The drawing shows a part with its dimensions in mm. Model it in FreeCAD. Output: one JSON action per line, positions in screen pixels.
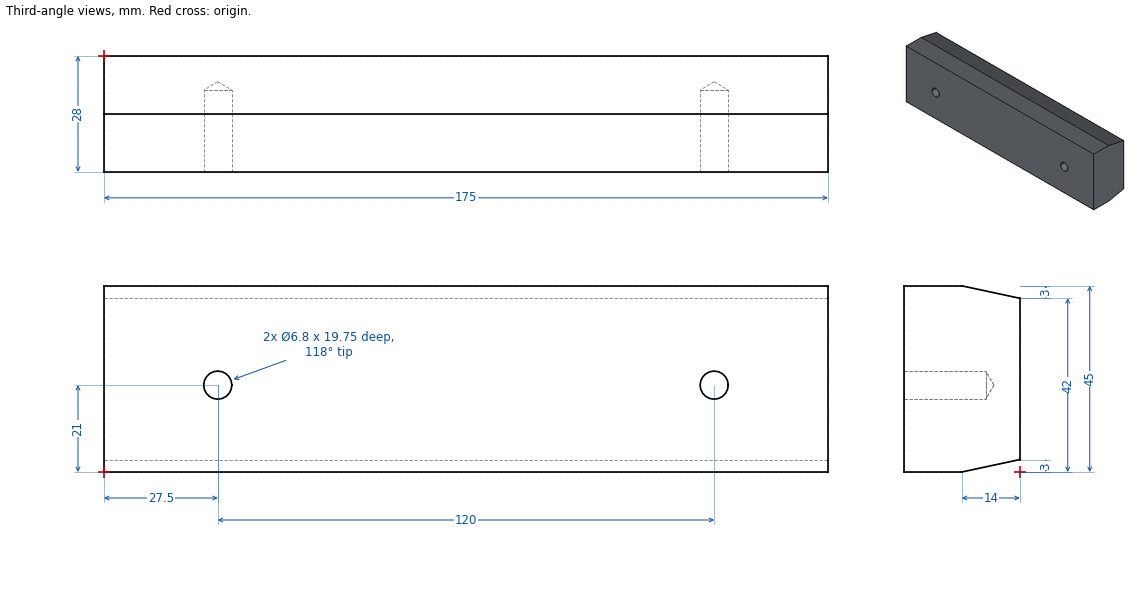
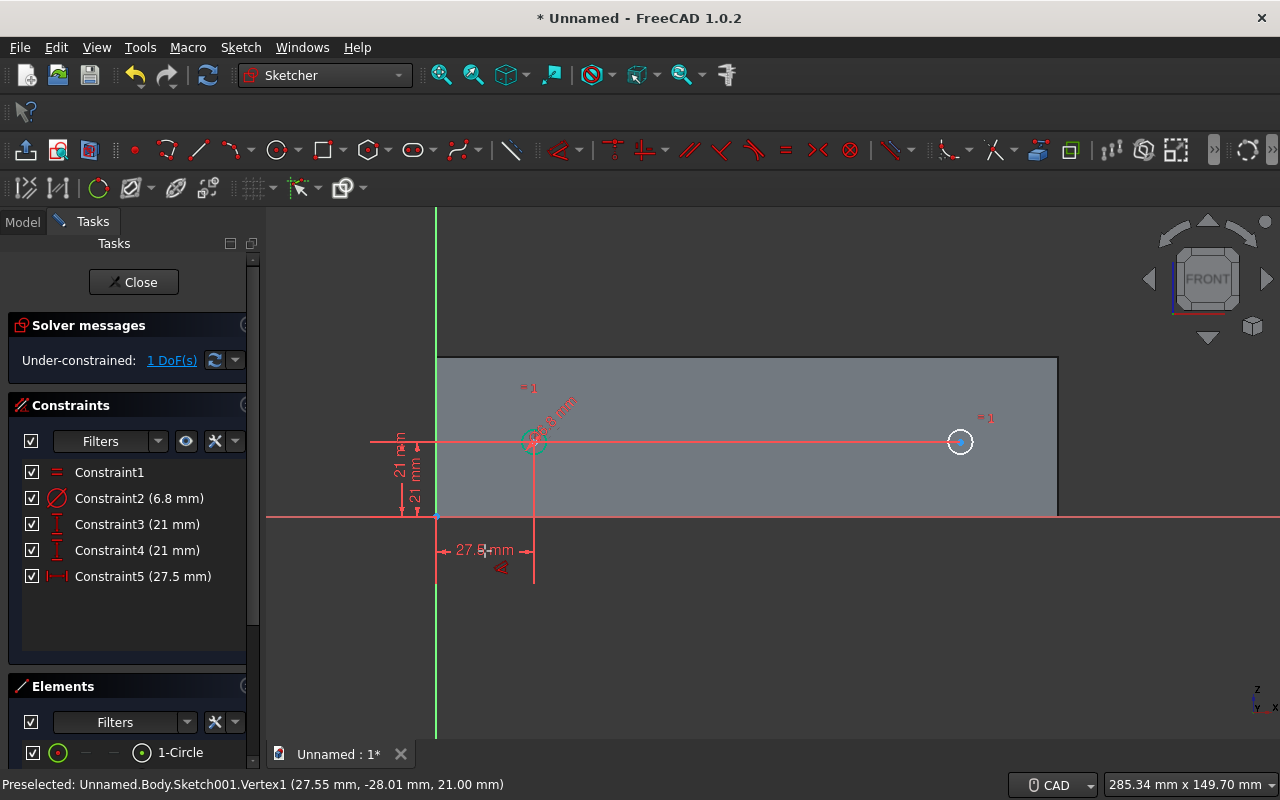
{"action": "left_click", "coordinate": [534, 442]}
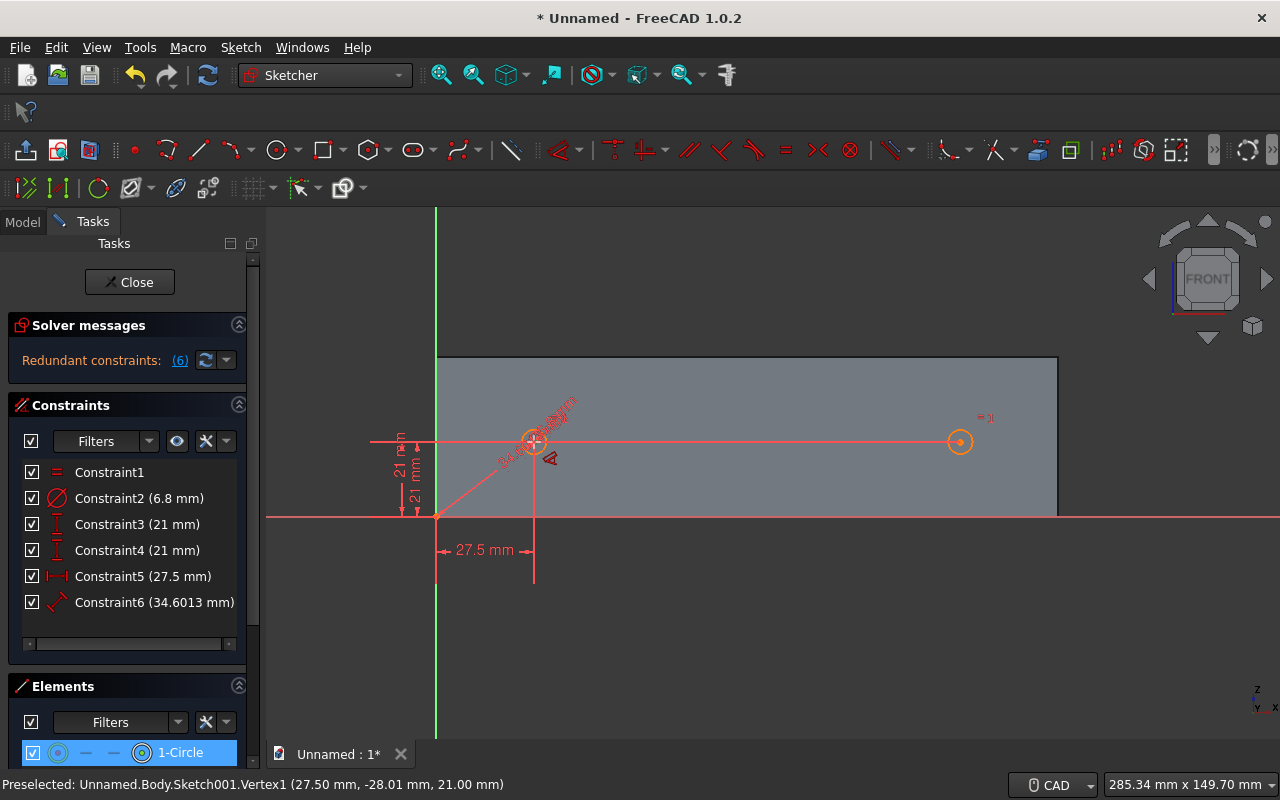
{"action": "left_click", "coordinate": [960, 442]}
{"action": "left_click", "coordinate": [747, 408]}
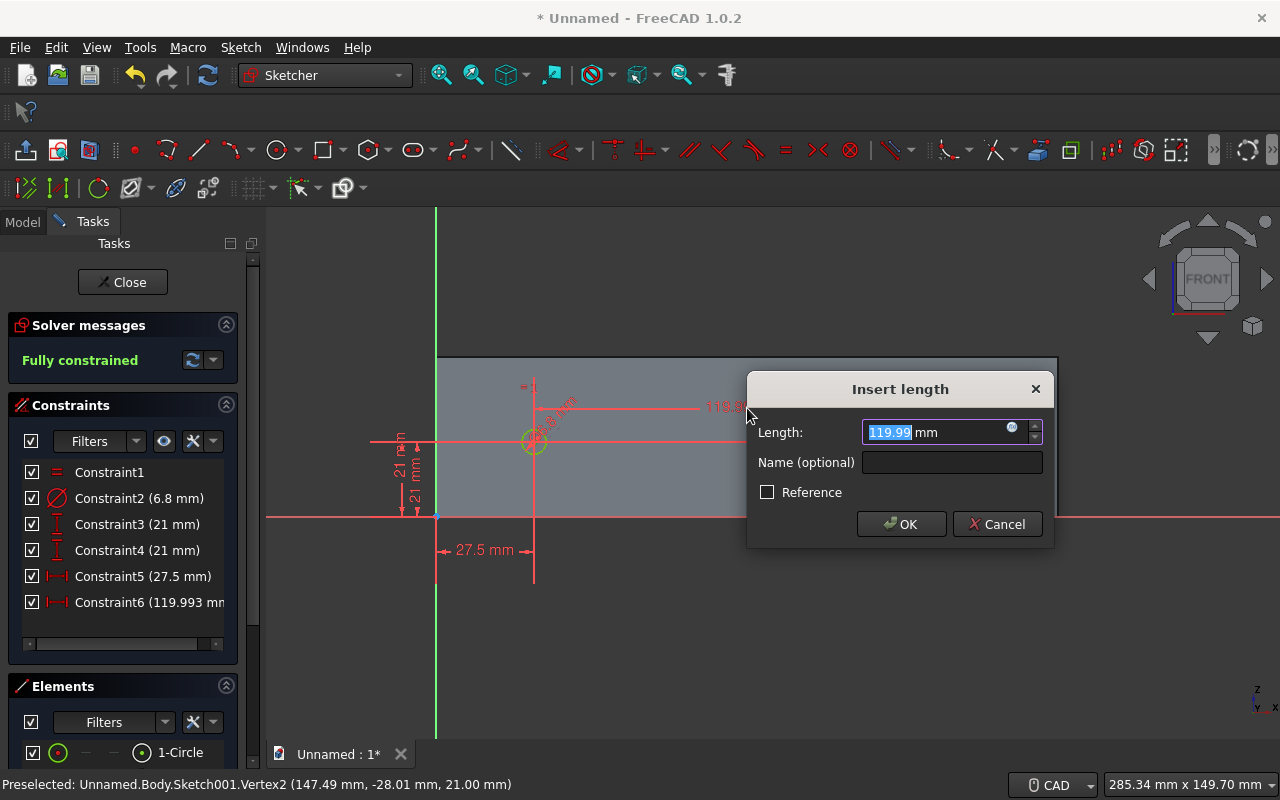
{"action": "type", "text": "120"}
{"action": "key", "text": "Return"}
{"action": "key", "text": "Escape"}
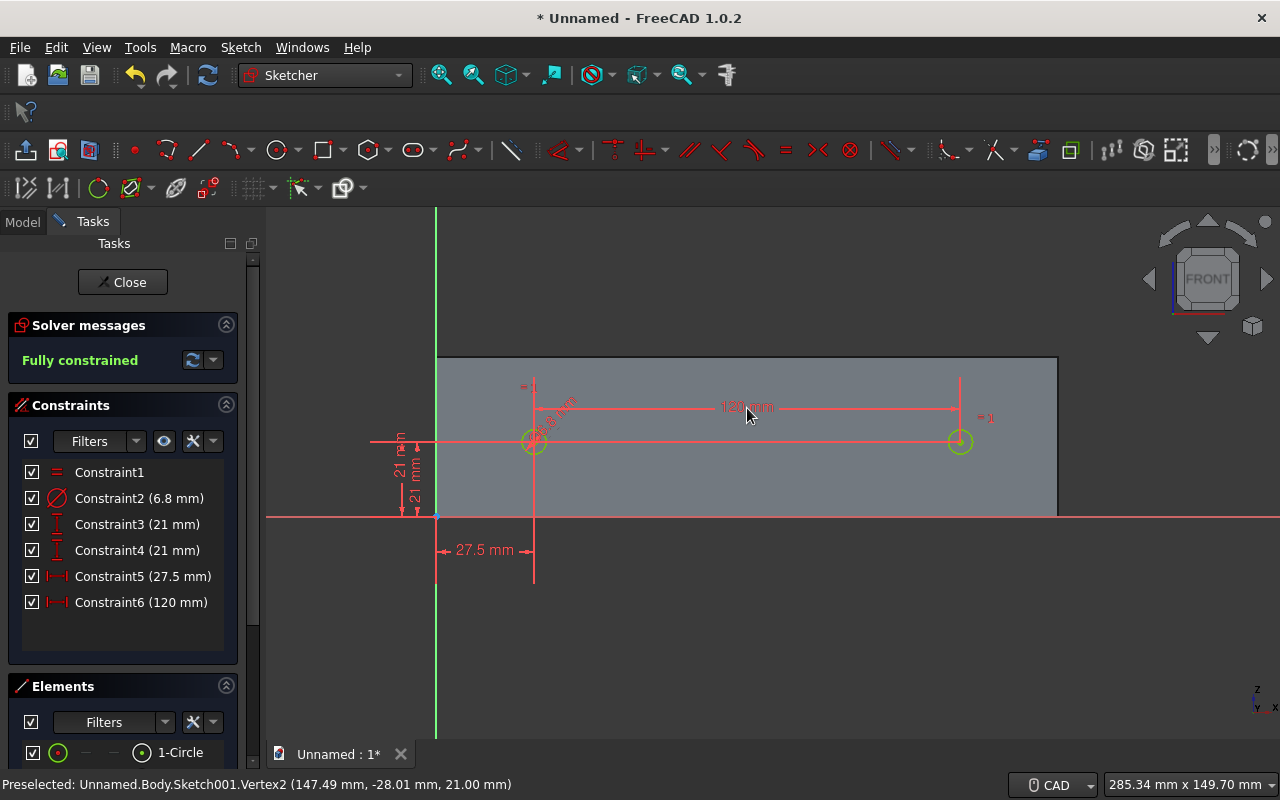
{"action": "left_click", "coordinate": [123, 282]}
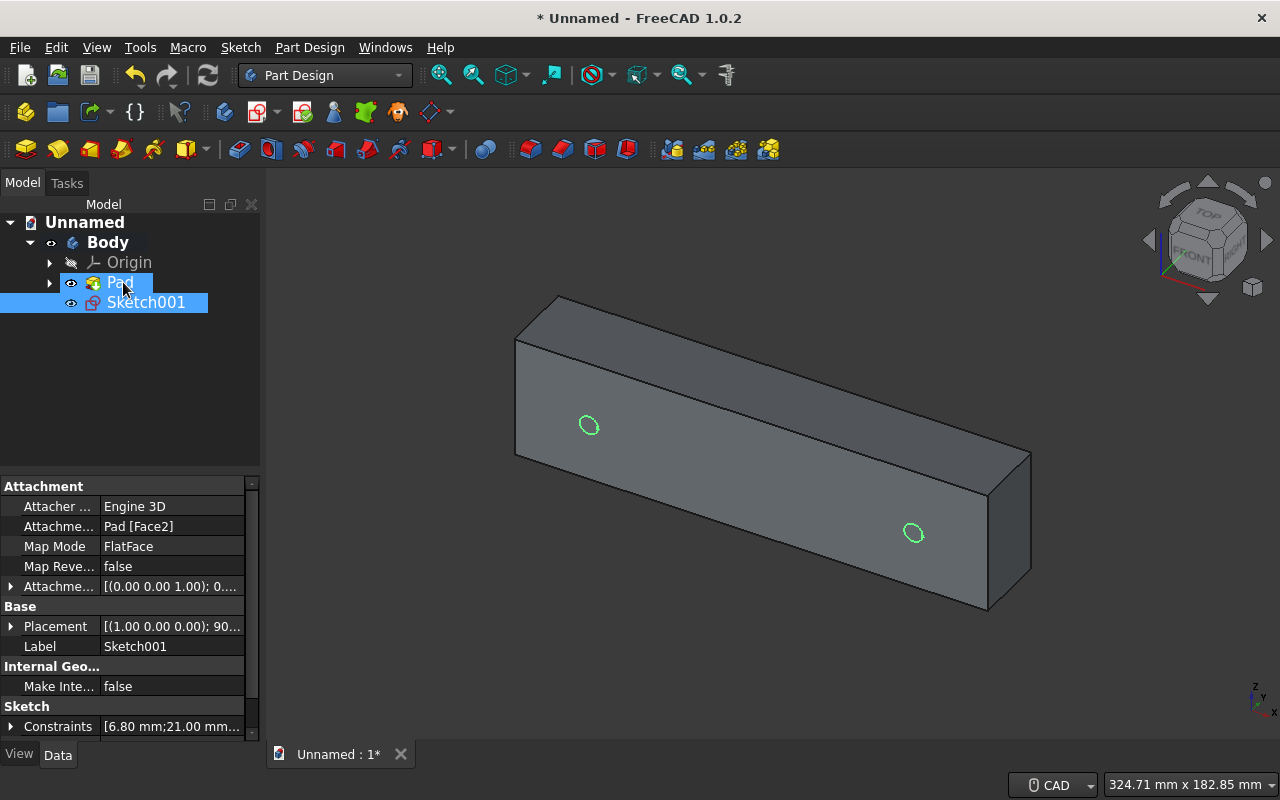
{"action": "left_click", "coordinate": [272, 150]}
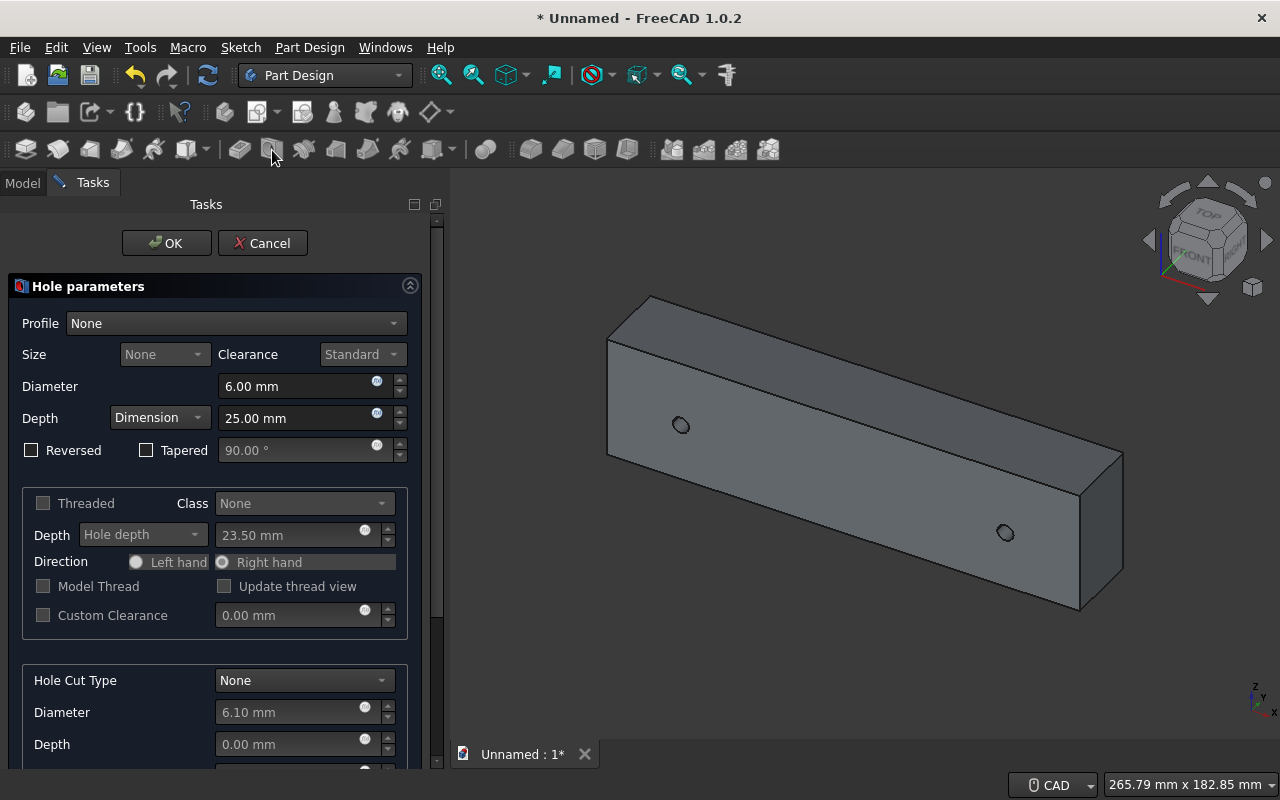
{"action": "triple_click", "coordinate": [305, 386]}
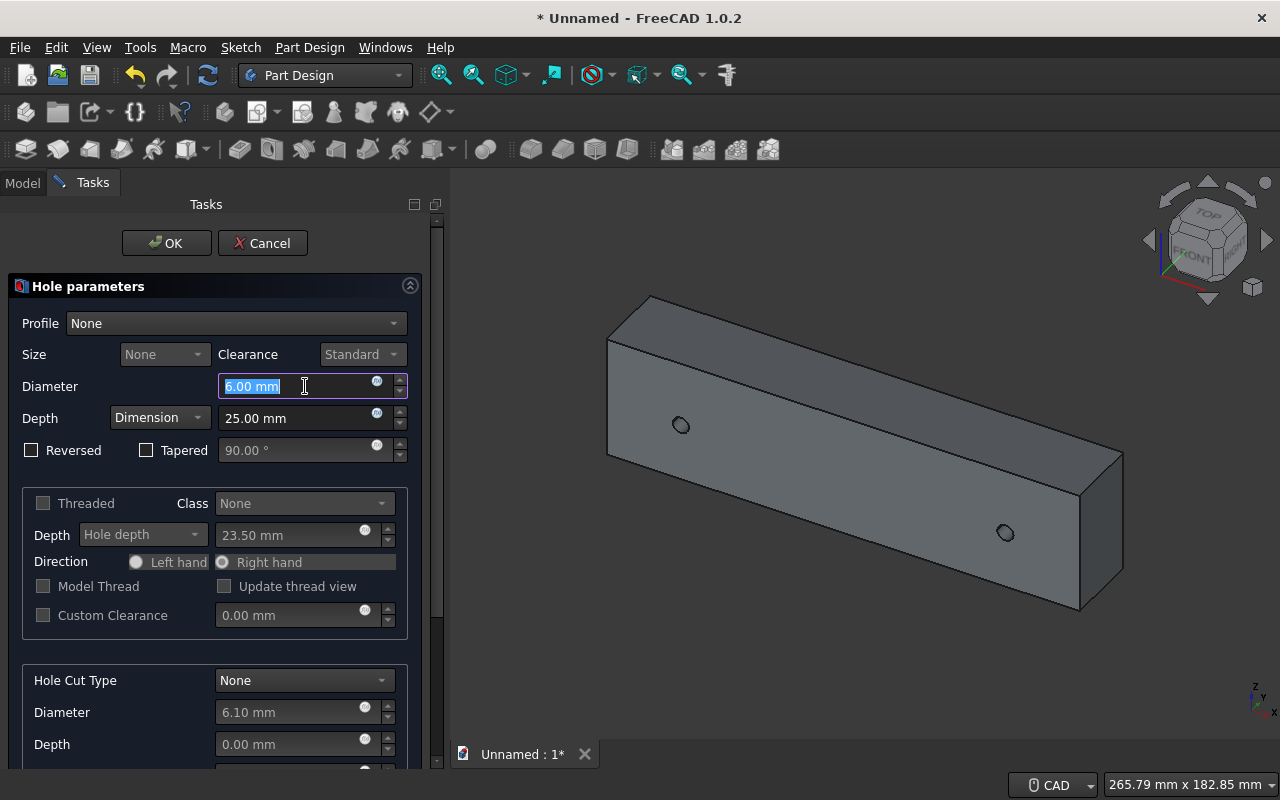
{"action": "type", "text": "6.8"}
{"action": "key", "text": "Tab"}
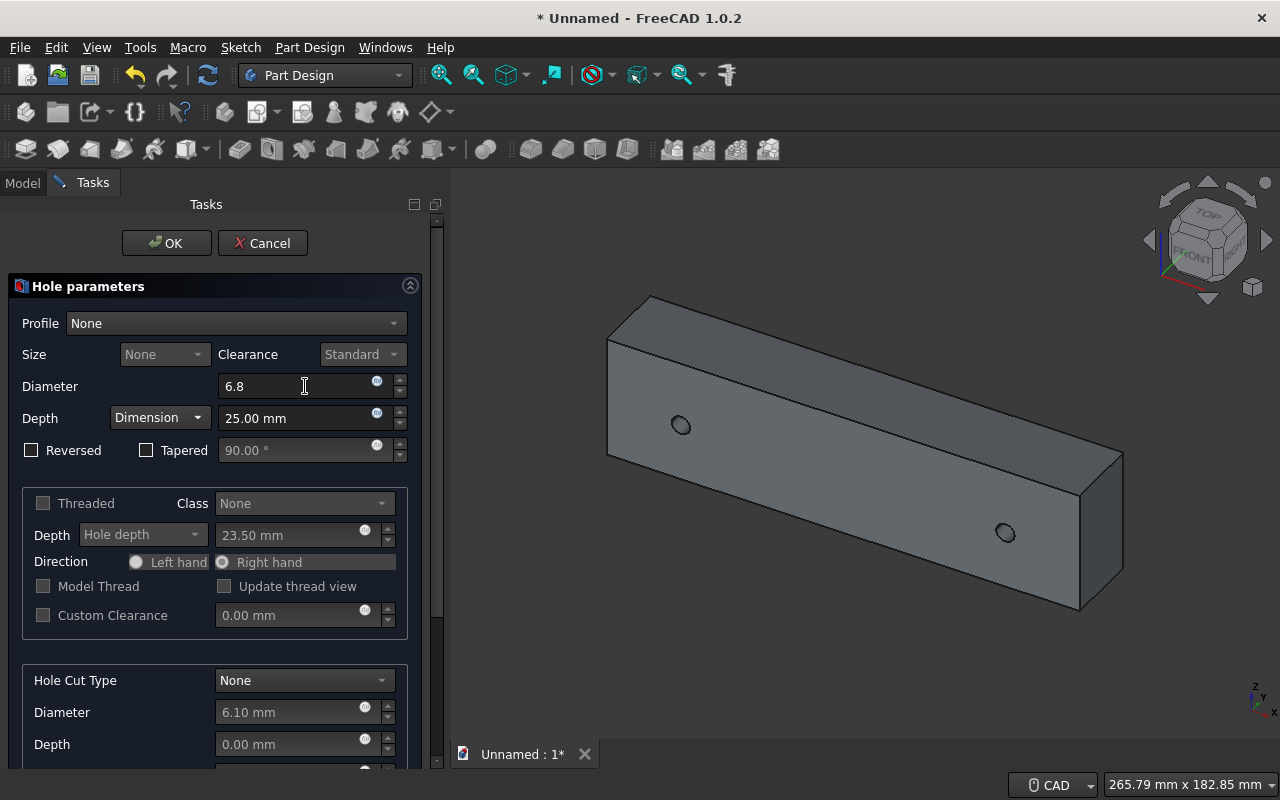
{"action": "triple_click", "coordinate": [305, 418]}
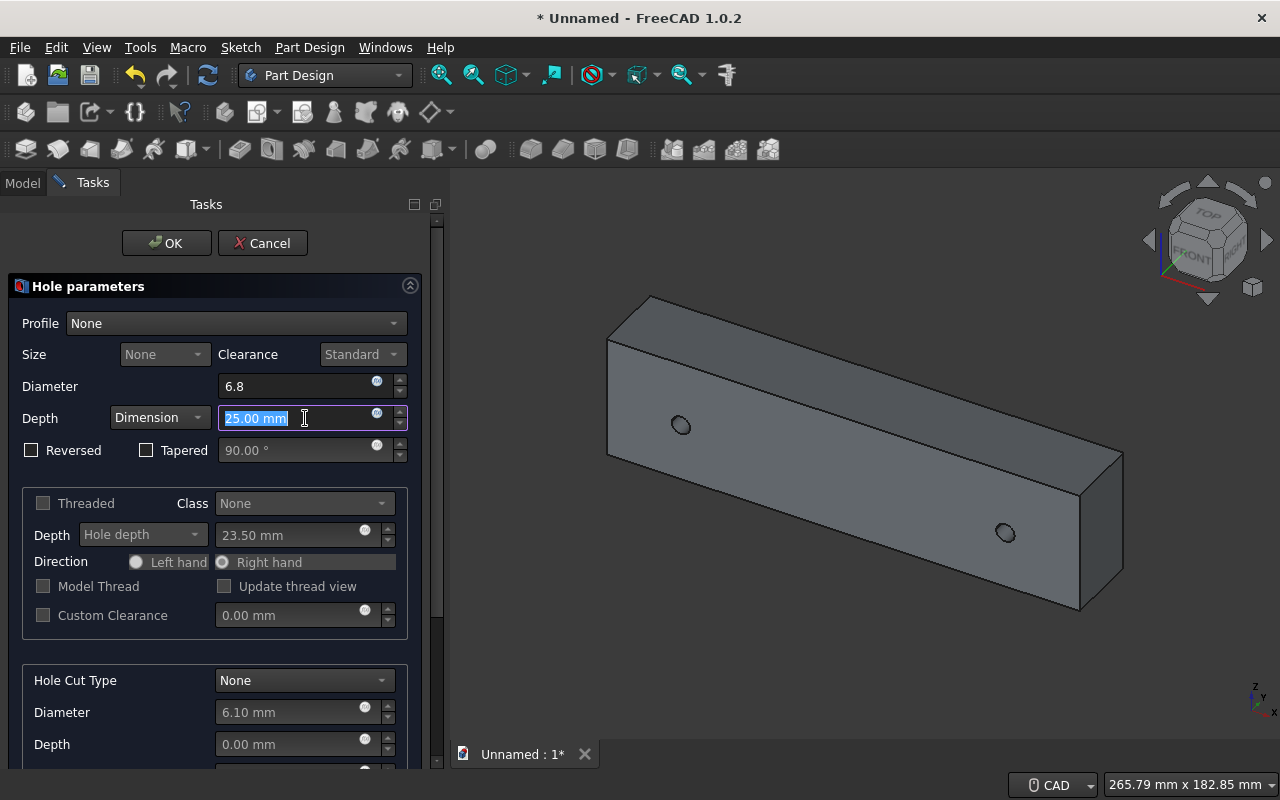
{"action": "type", "text": "19.75"}
{"action": "key", "text": "Tab"}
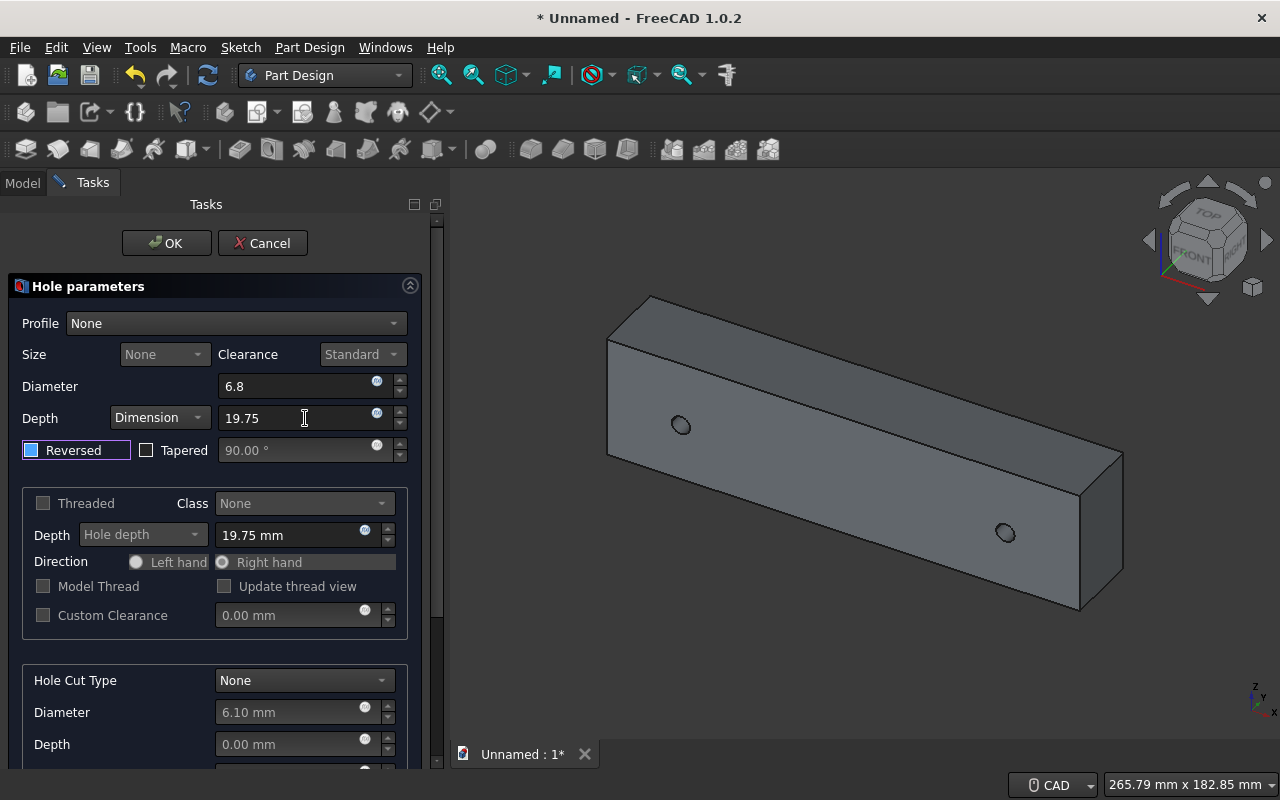
{"action": "left_click", "coordinate": [167, 243]}